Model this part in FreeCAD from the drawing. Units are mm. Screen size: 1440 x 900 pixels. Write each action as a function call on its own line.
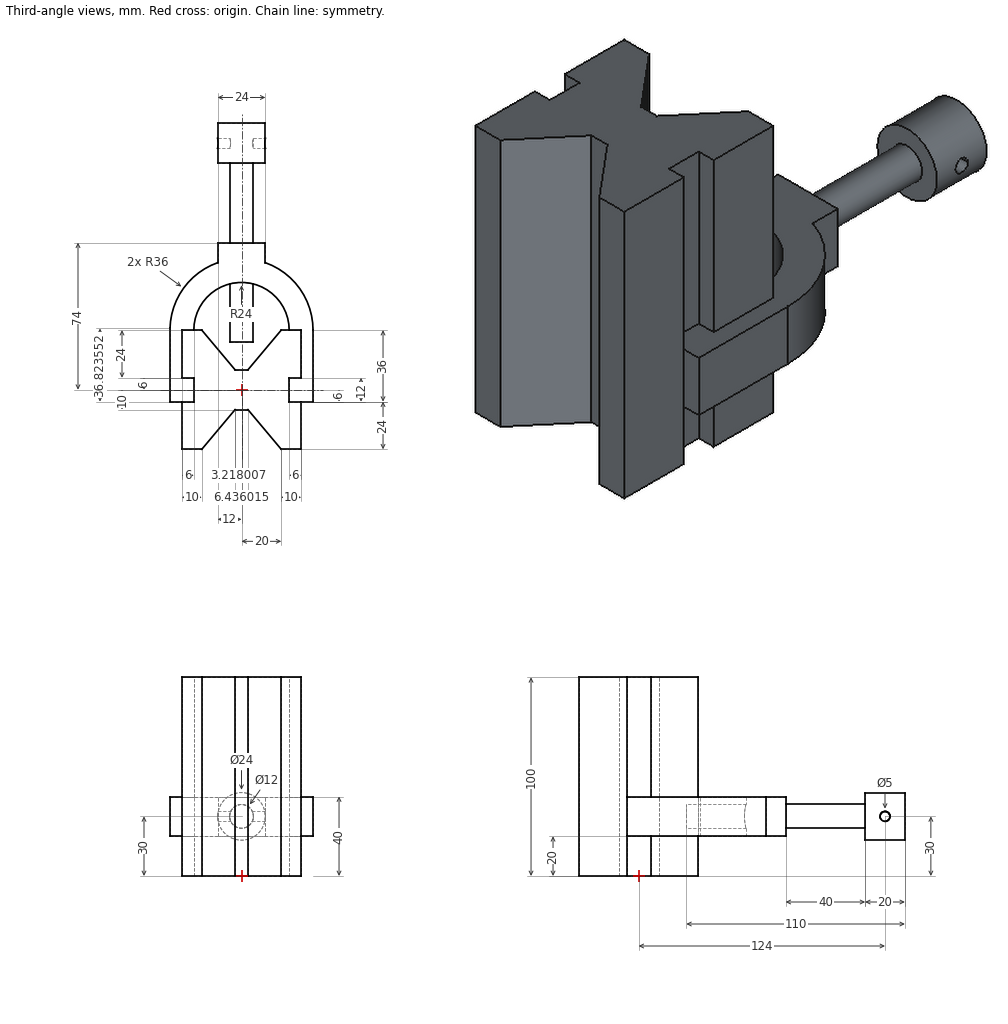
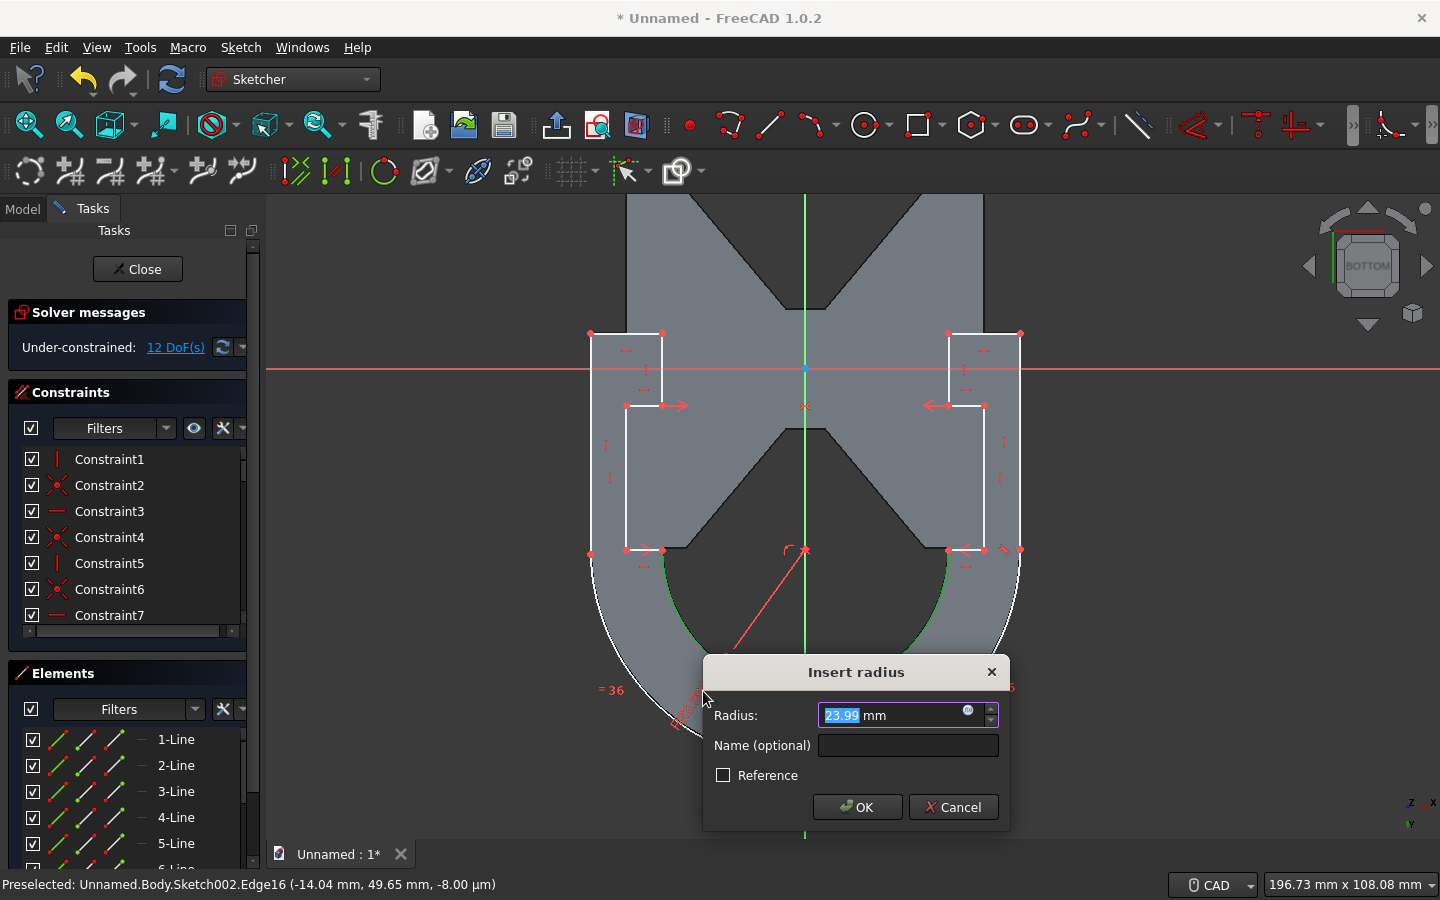
text(24)
key(Return)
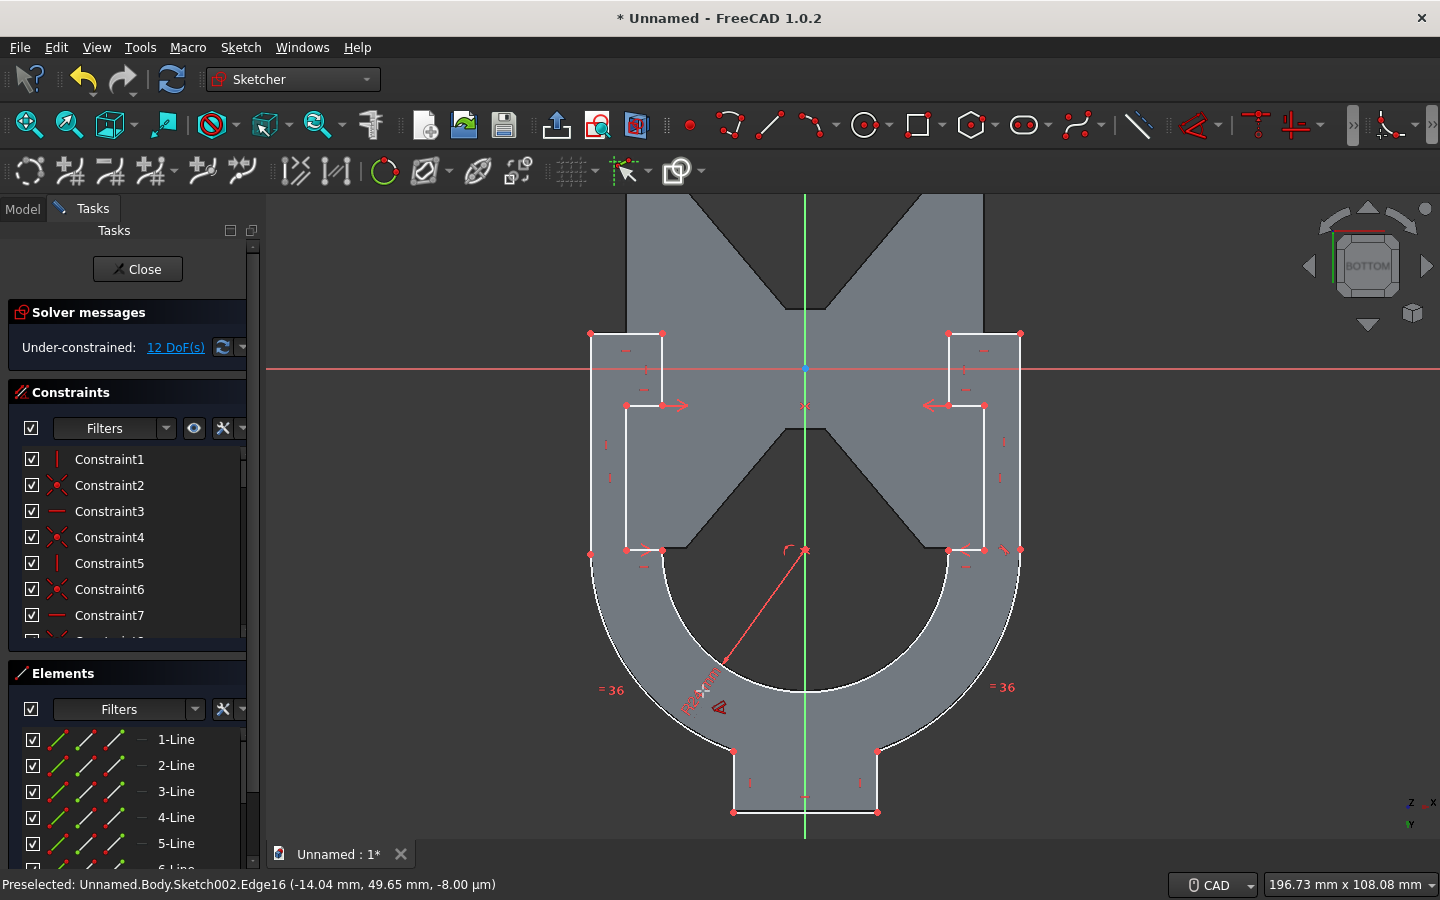
click(607, 630)
click(577, 642)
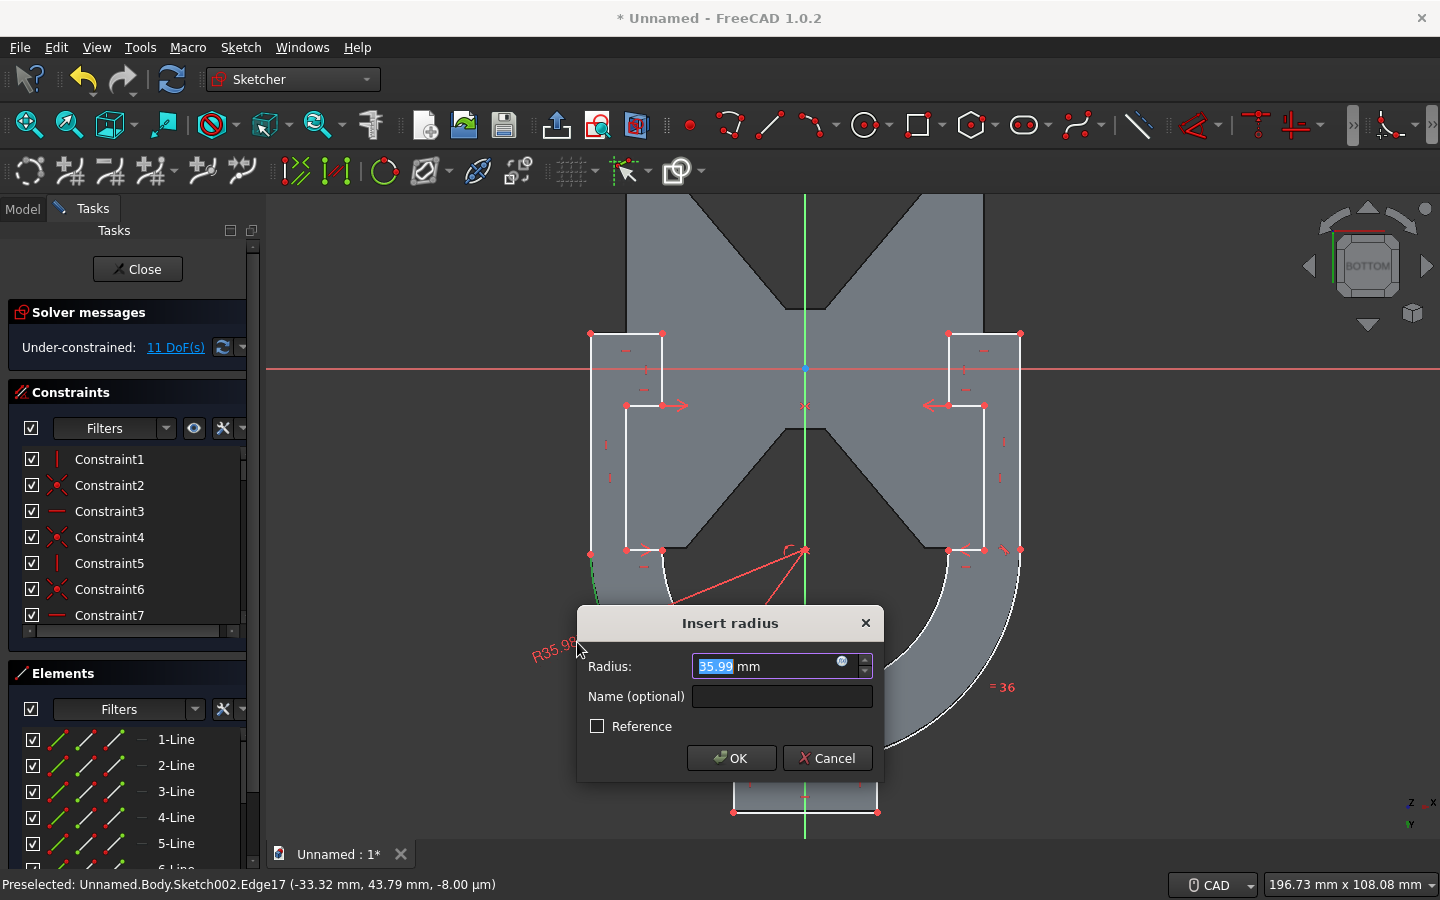
text(36)
key(Return)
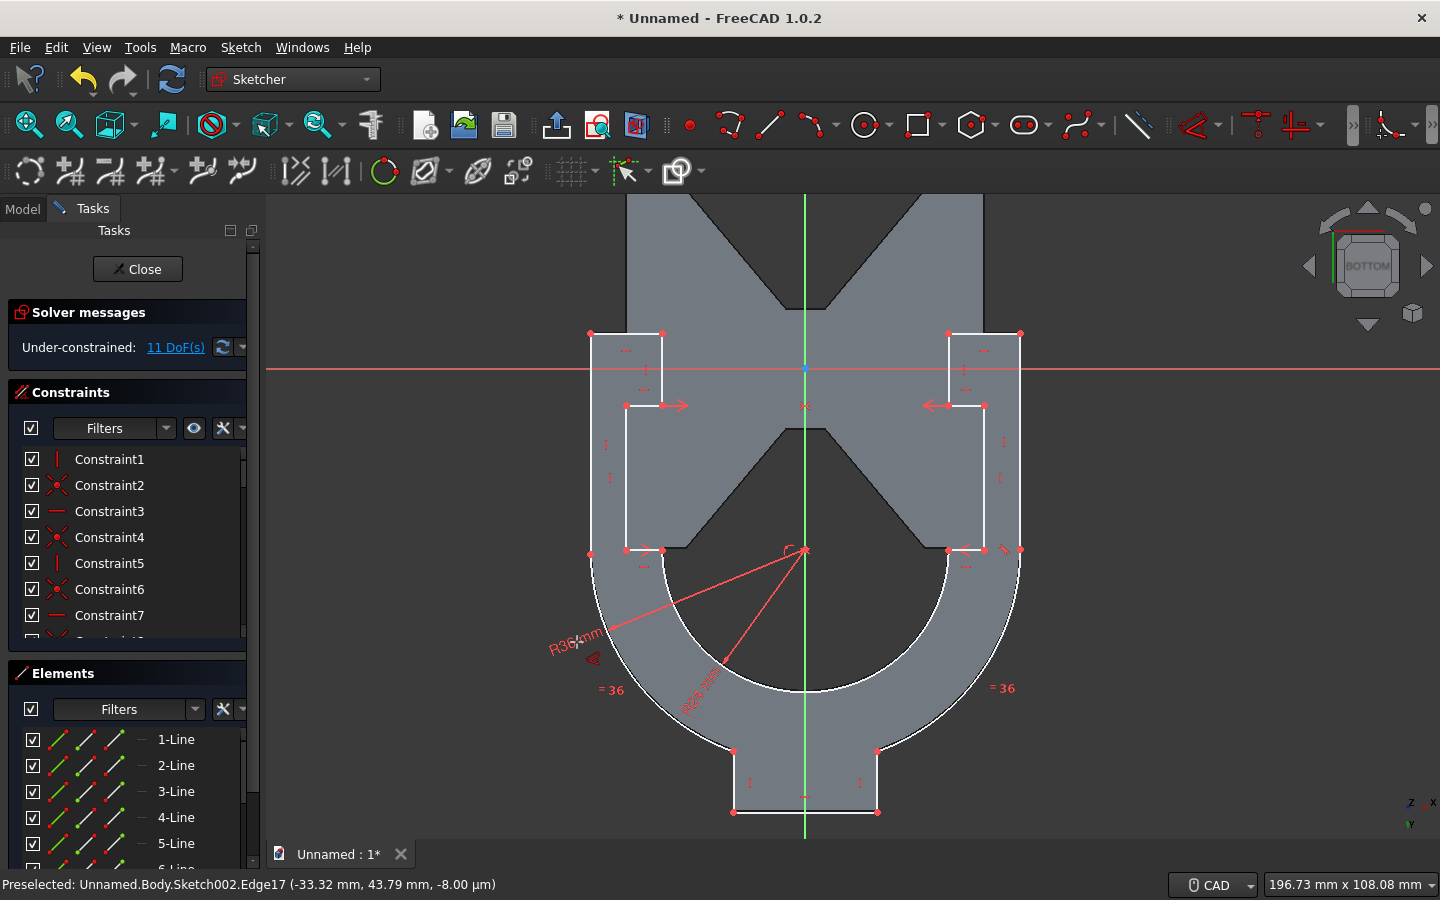
scroll(959, 406, up, 2)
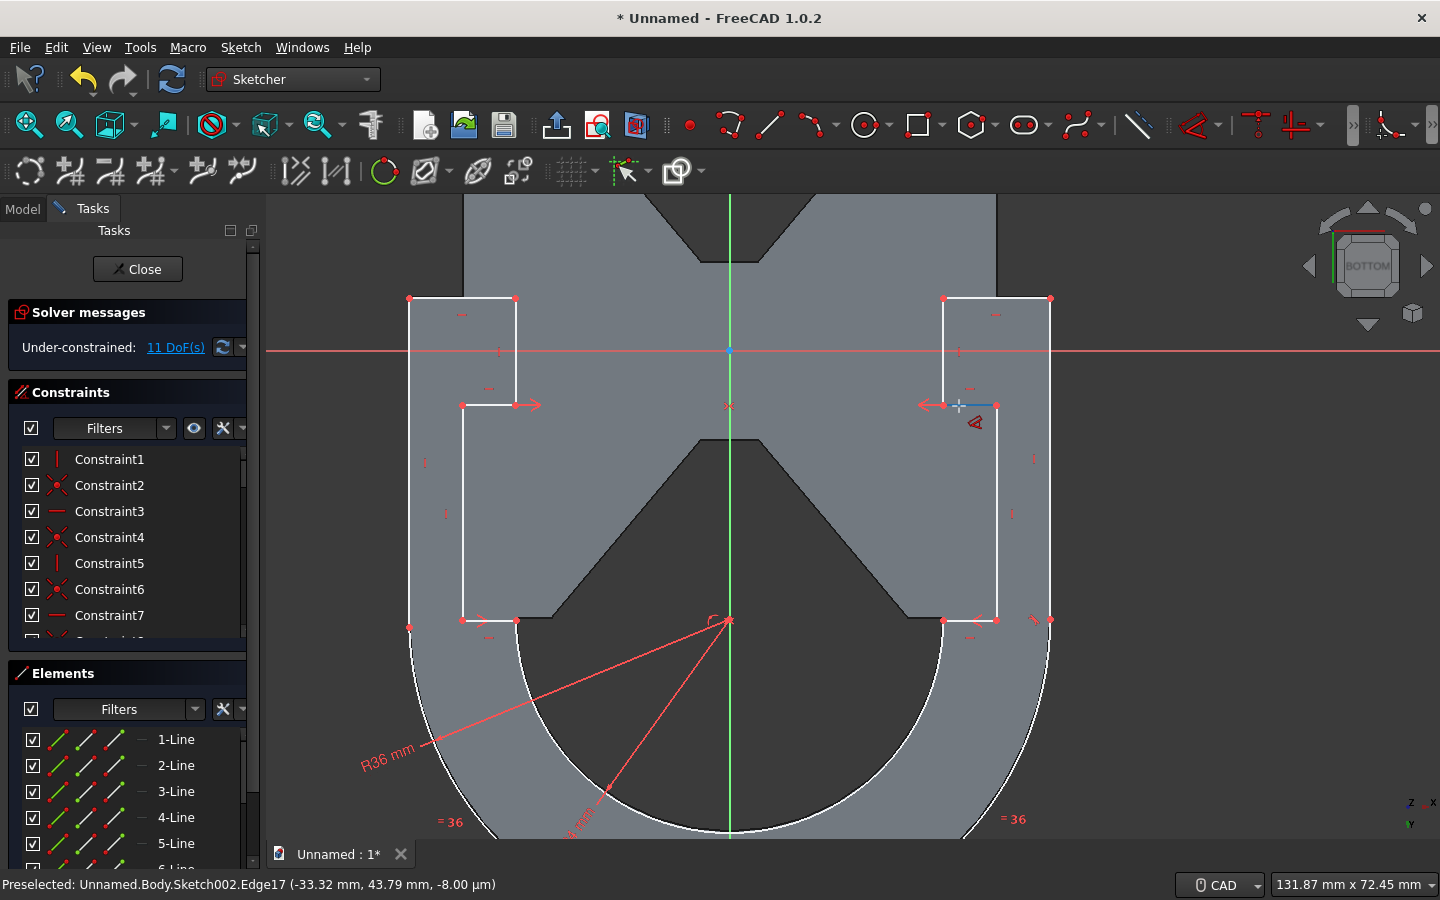
click(959, 405)
click(970, 371)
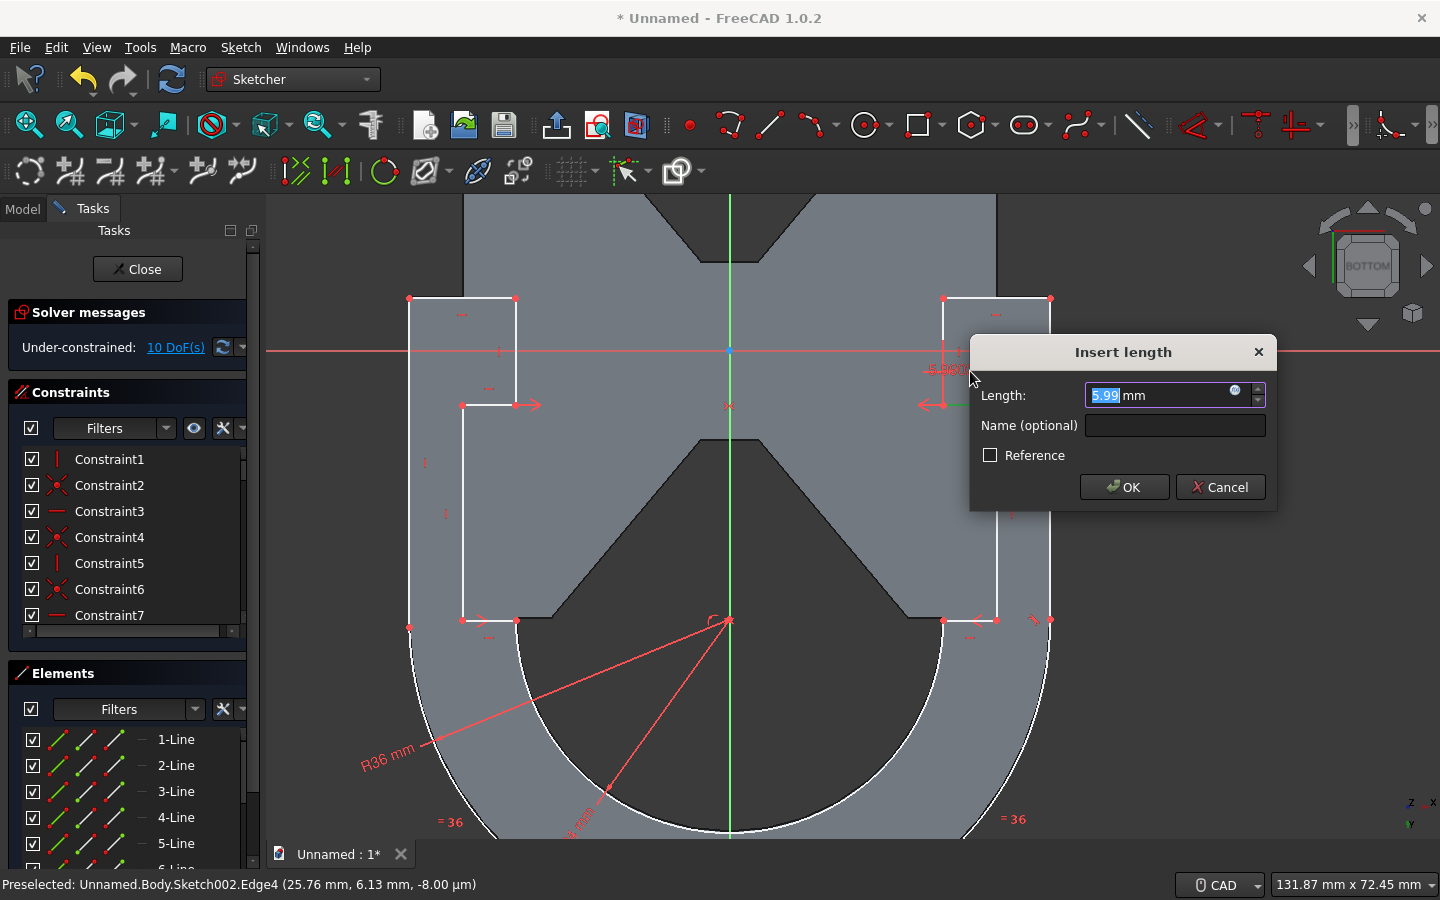
text(6)
key(Return)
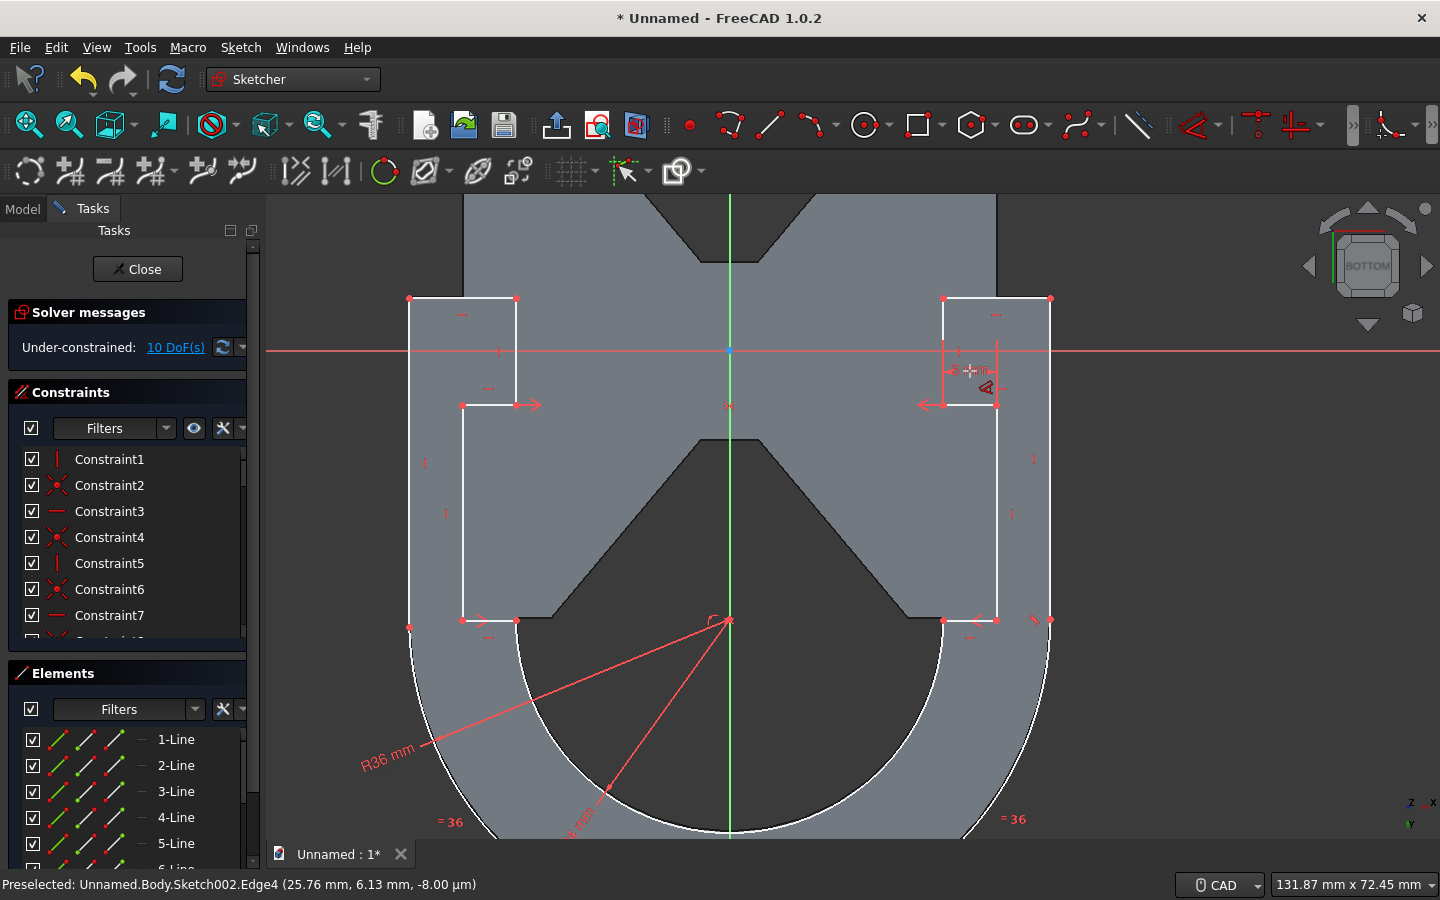
click(981, 621)
click(970, 587)